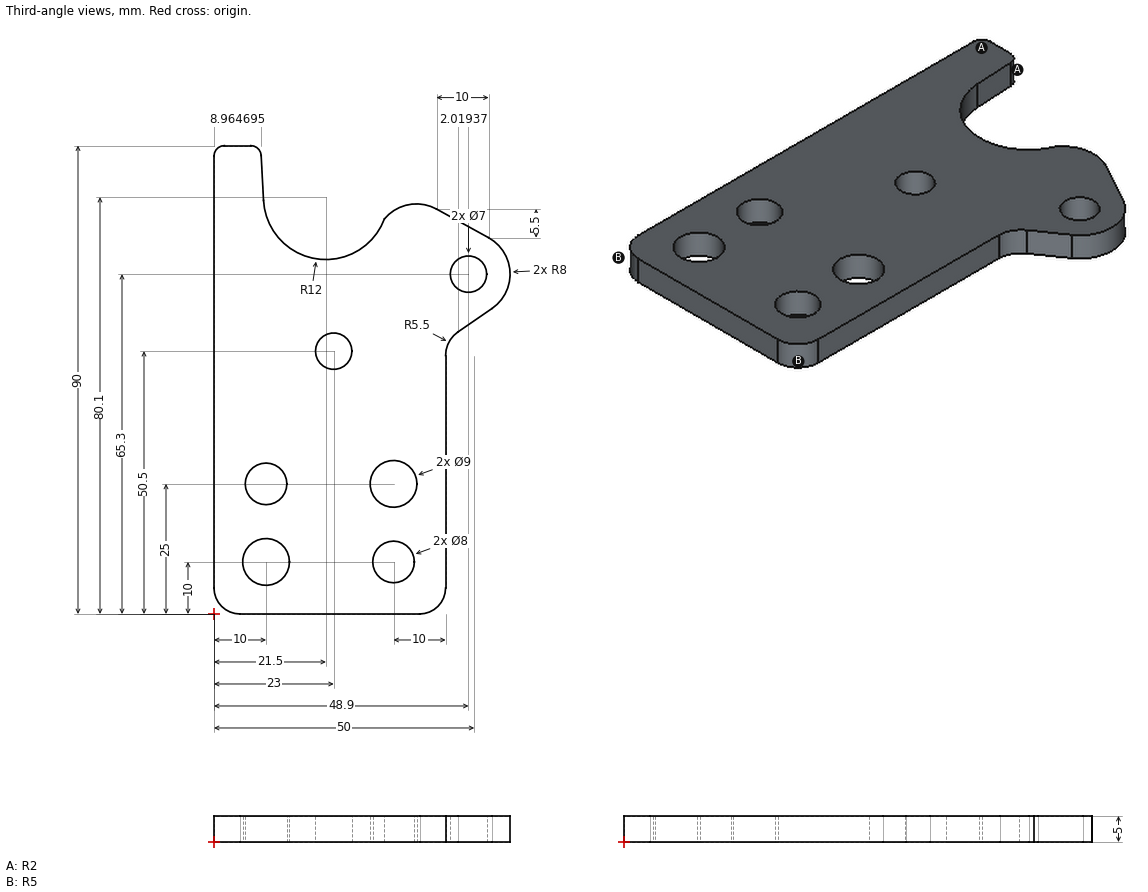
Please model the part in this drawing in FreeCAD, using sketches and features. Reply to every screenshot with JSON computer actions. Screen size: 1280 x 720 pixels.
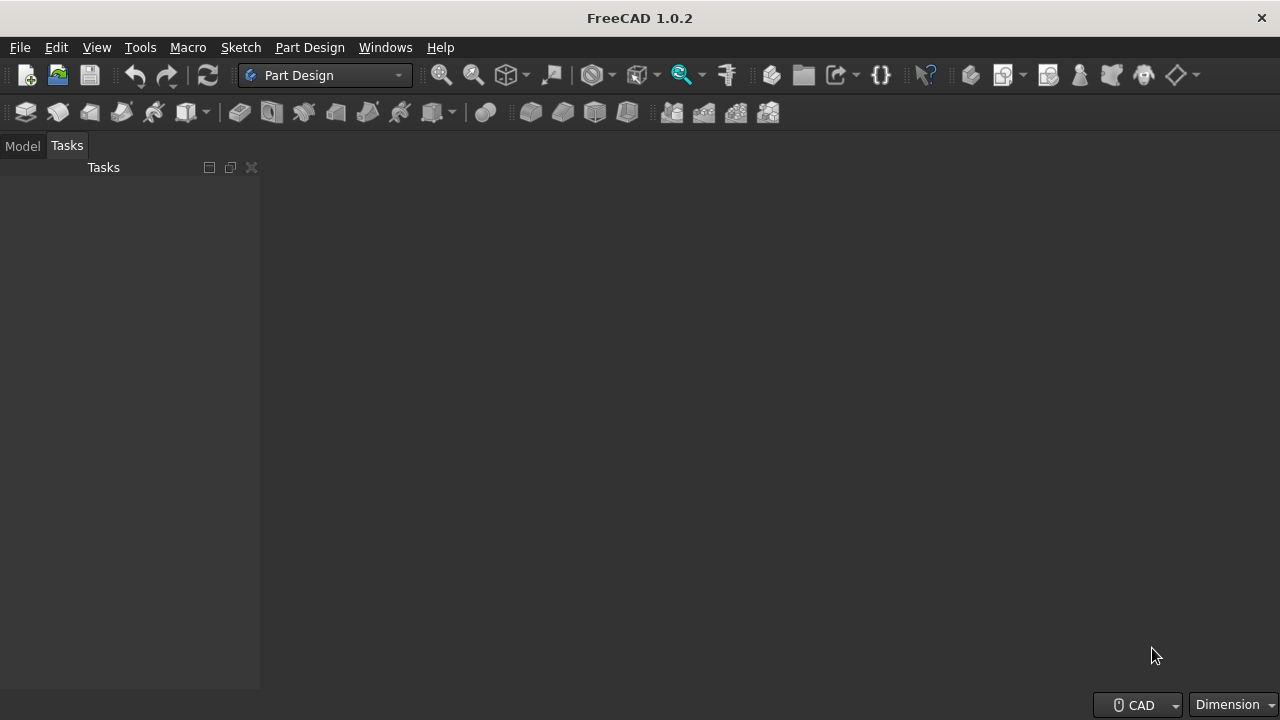
{"action": "left_click", "coordinate": [26, 76]}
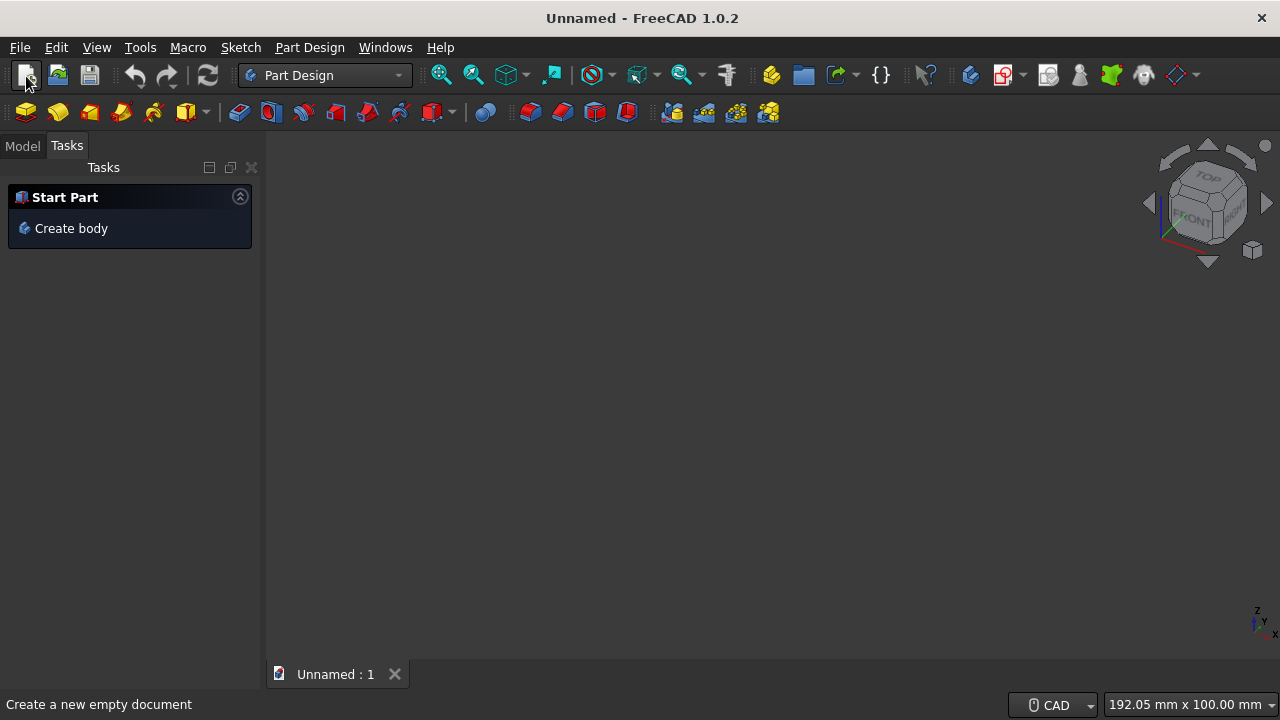
{"action": "left_click", "coordinate": [1004, 76]}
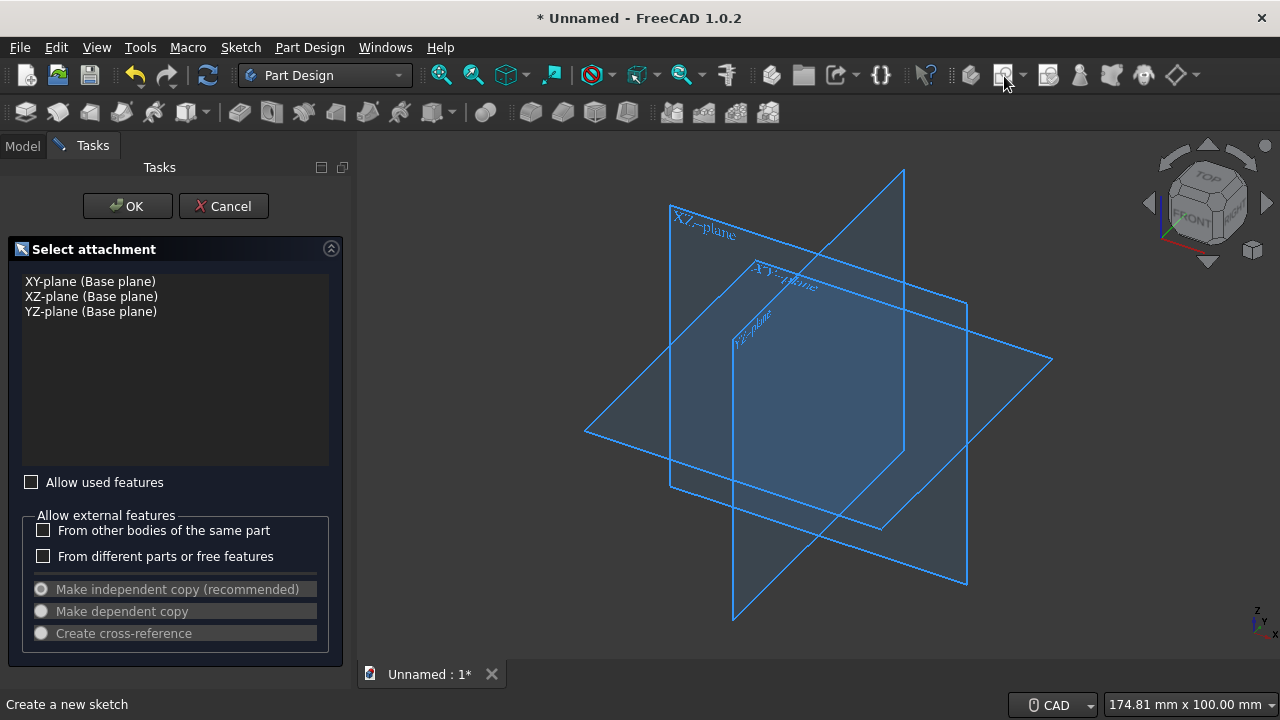
{"action": "left_click", "coordinate": [82, 282]}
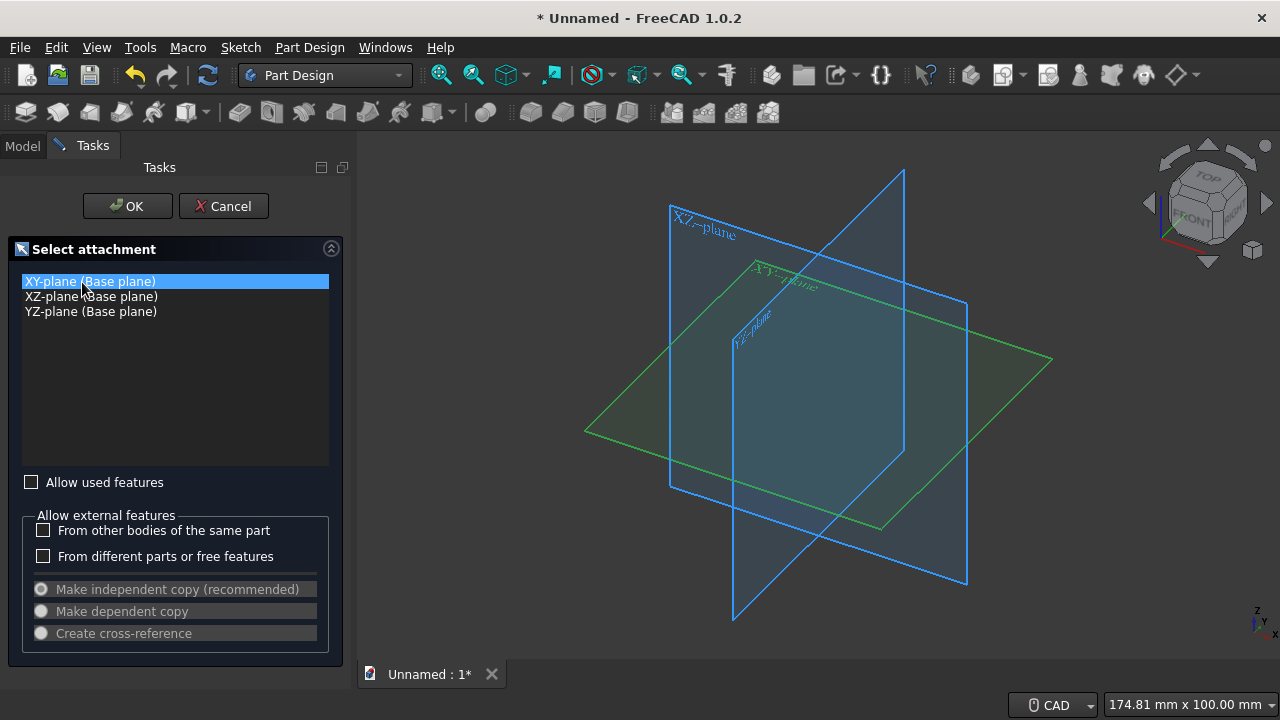
{"action": "left_click", "coordinate": [128, 206]}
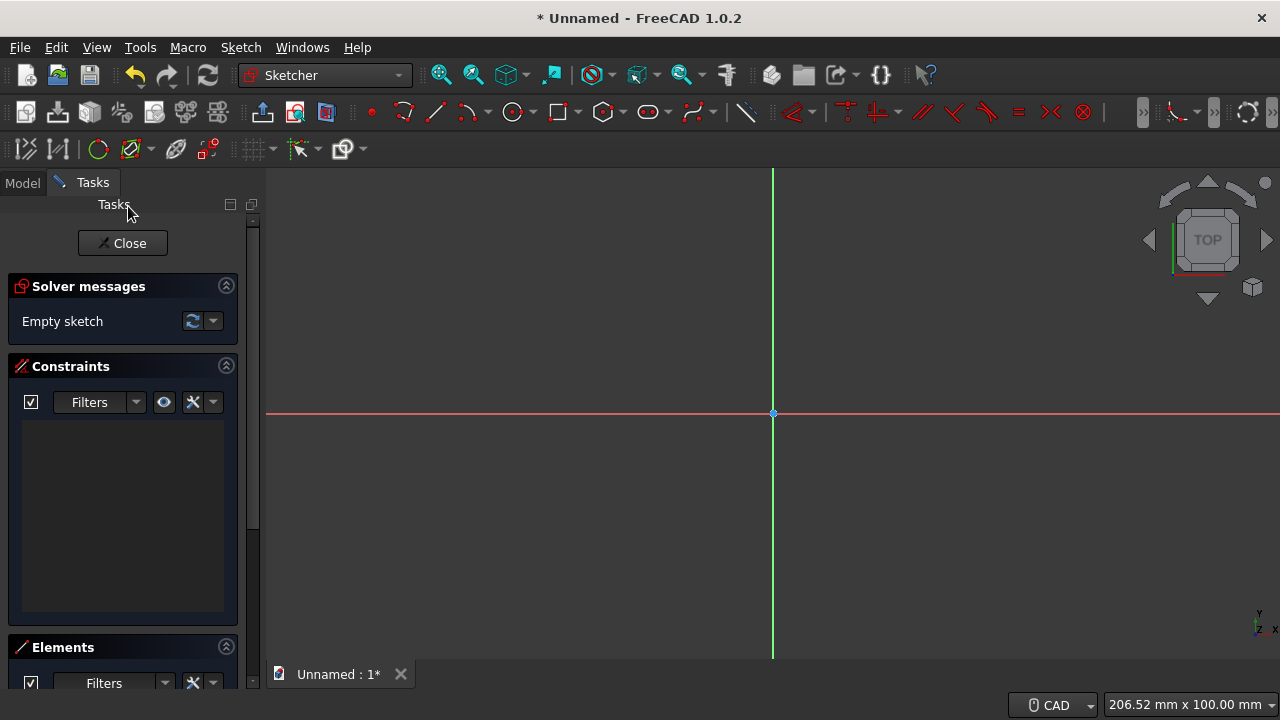
{"action": "scroll", "coordinate": [451, 631], "scroll_direction": "down", "scroll_amount": 3}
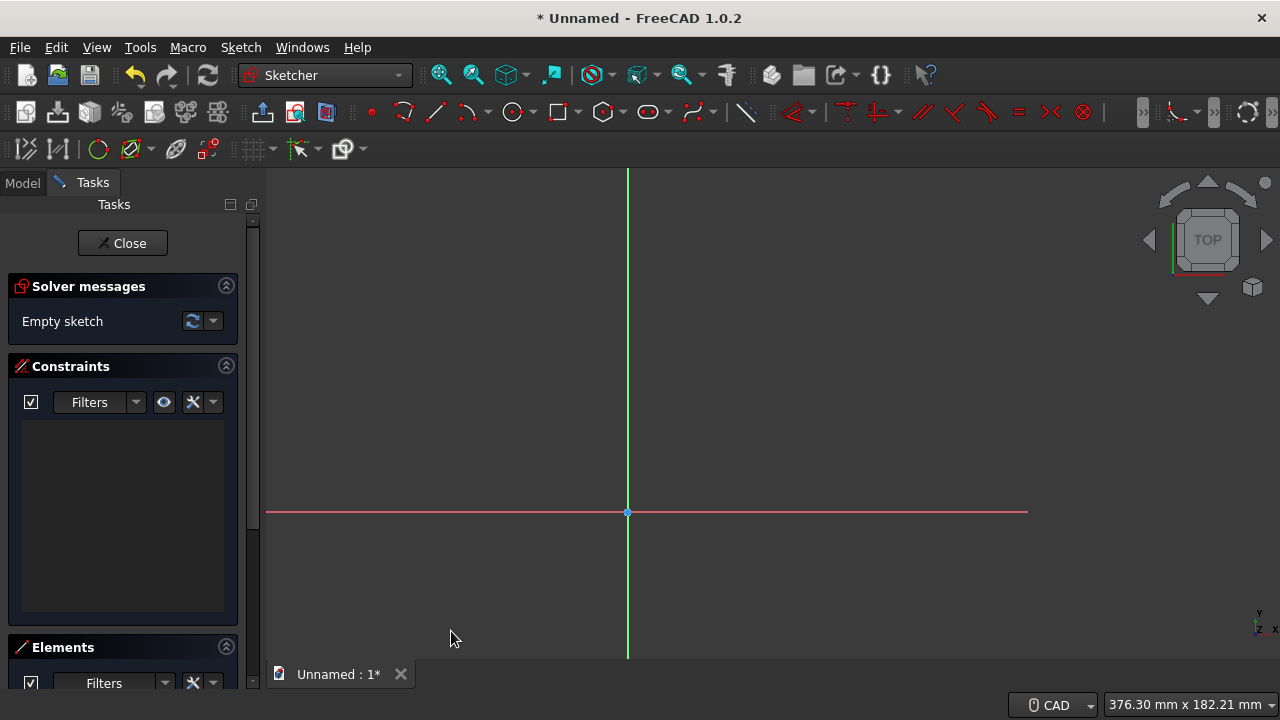
{"action": "key", "text": "g m"}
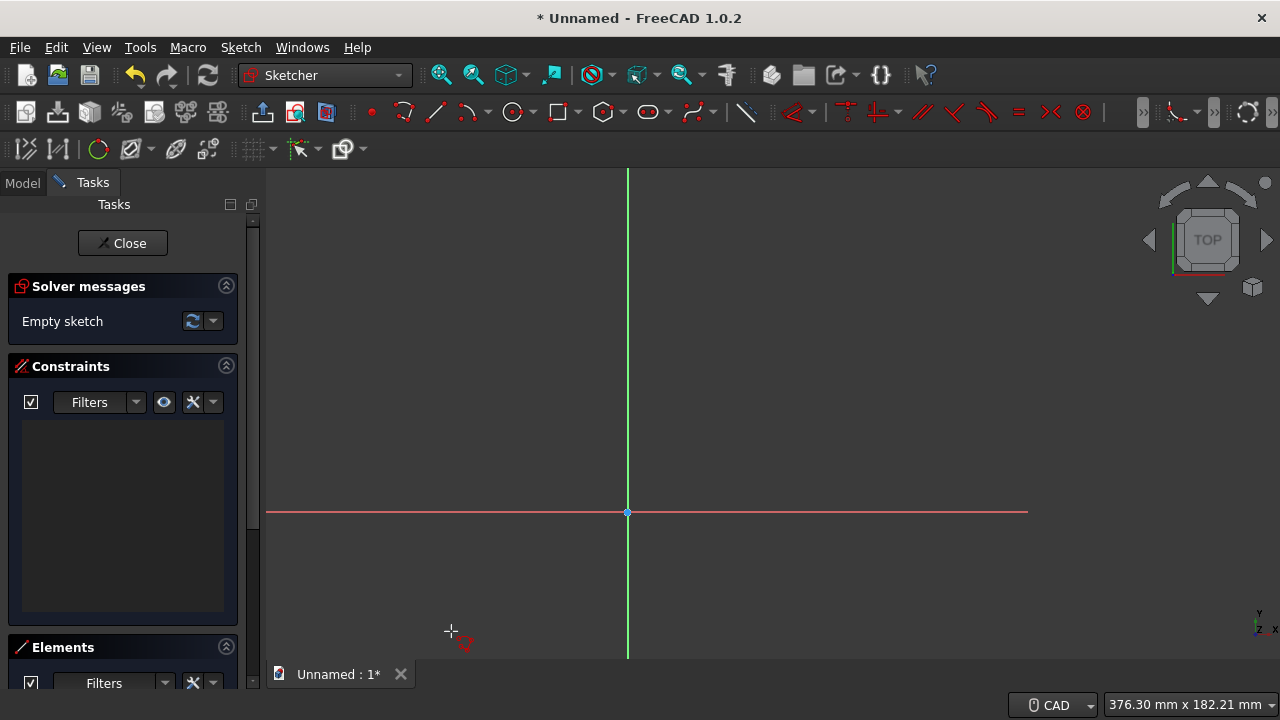
{"action": "left_click", "coordinate": [653, 298]}
{"action": "left_click", "coordinate": [650, 270]}
{"action": "left_click", "coordinate": [628, 270]}
{"action": "left_click", "coordinate": [628, 512]}
{"action": "left_click", "coordinate": [748, 503]}
{"action": "left_click", "coordinate": [748, 378]}
{"action": "right_click", "coordinate": [748, 378]}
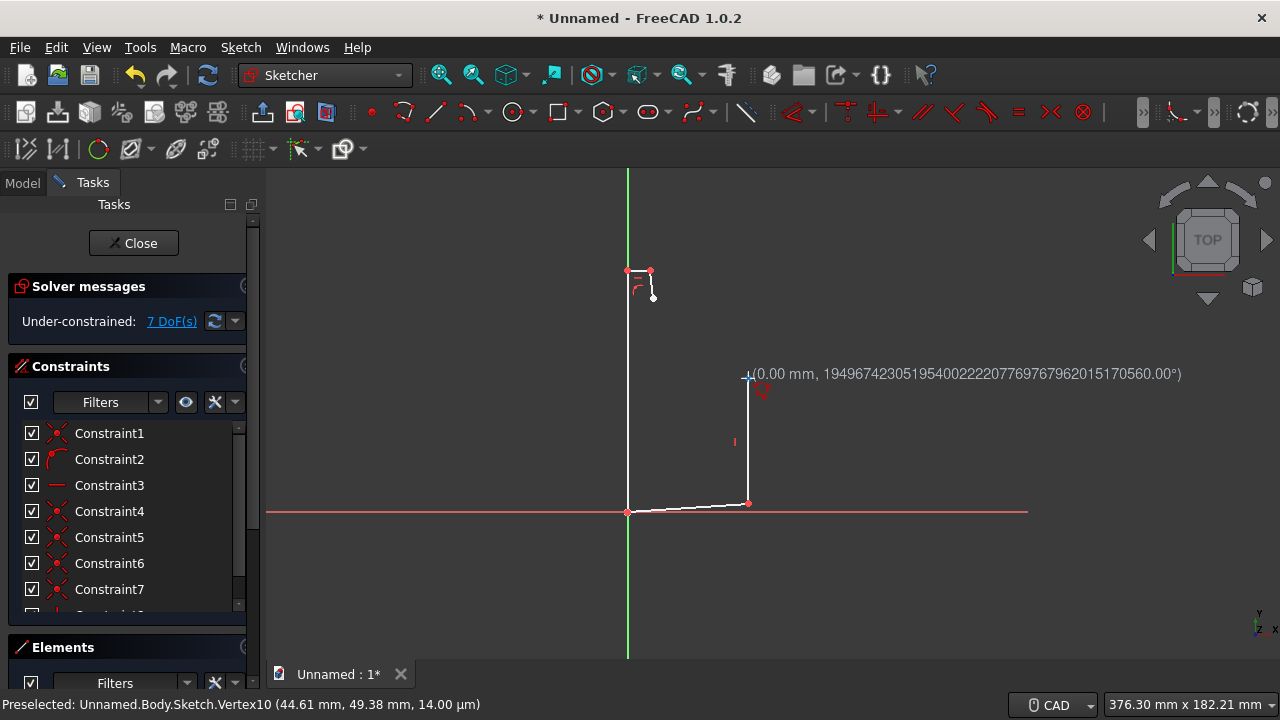
{"action": "key", "text": "g l"}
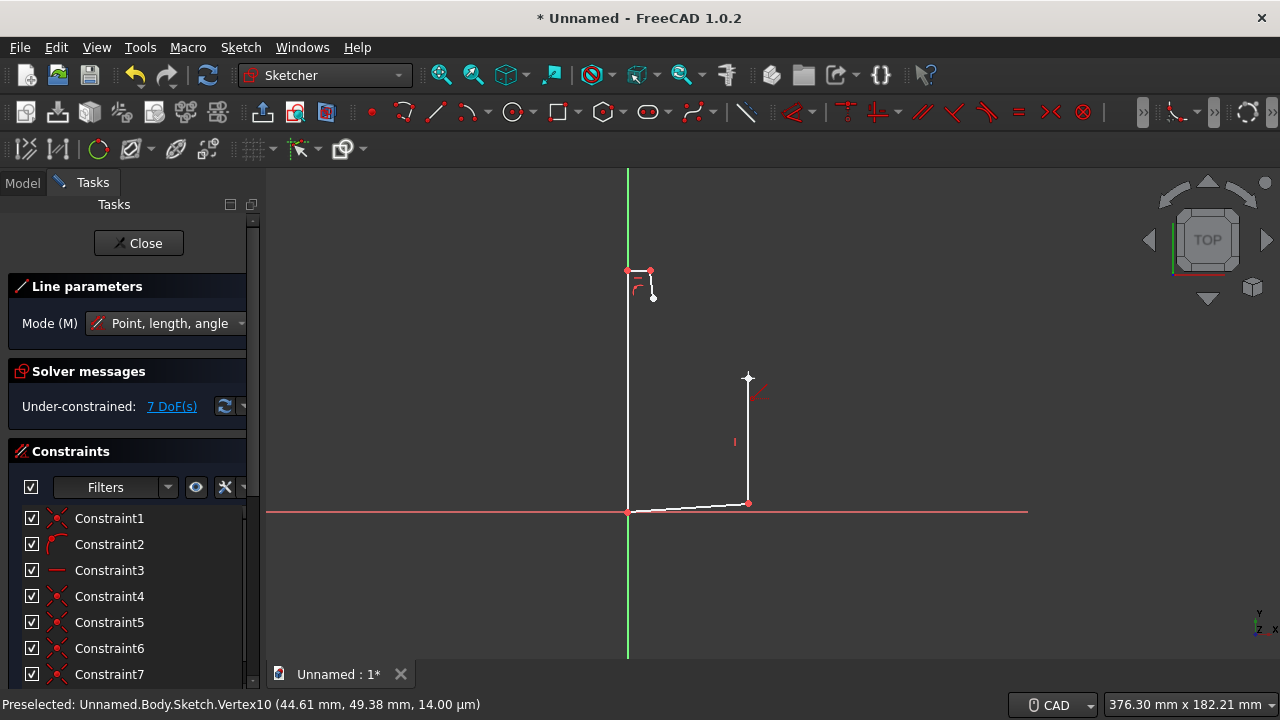
{"action": "left_click", "coordinate": [754, 366]}
{"action": "left_click", "coordinate": [772, 354]}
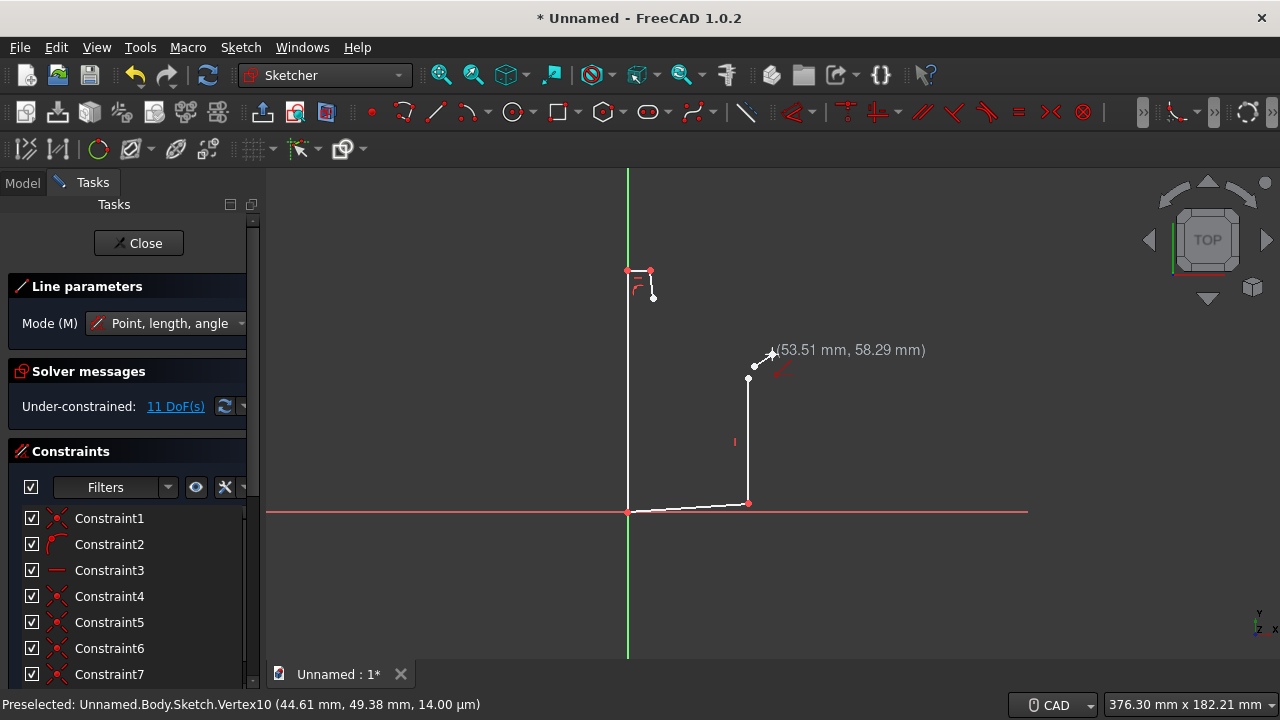
{"action": "left_click", "coordinate": [770, 317]}
{"action": "left_click", "coordinate": [743, 302]}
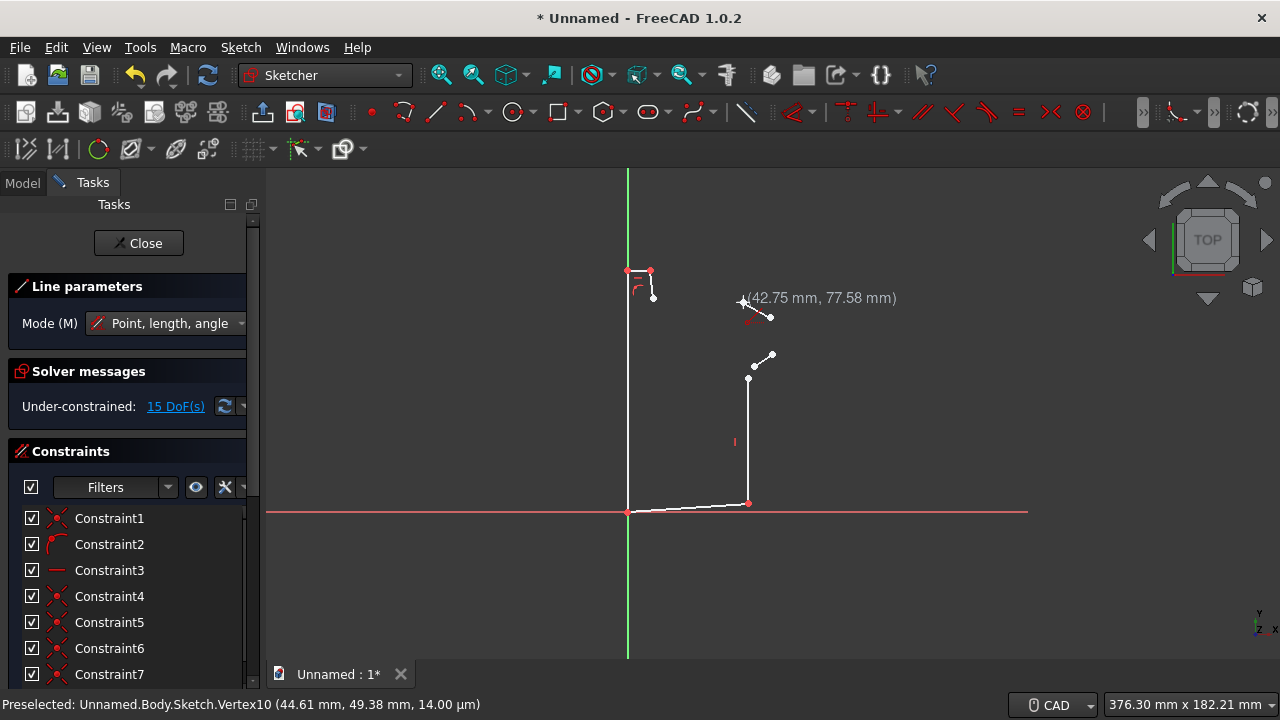
{"action": "key", "text": "g 3 a"}